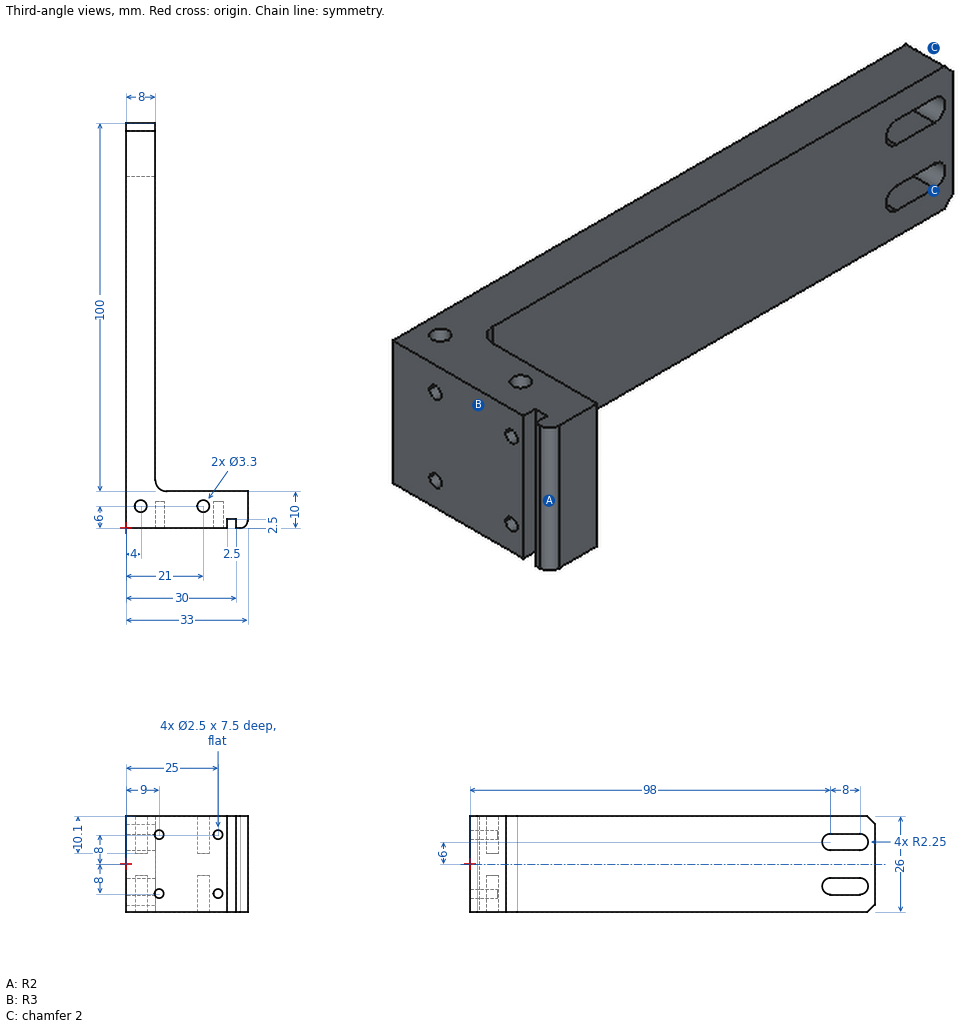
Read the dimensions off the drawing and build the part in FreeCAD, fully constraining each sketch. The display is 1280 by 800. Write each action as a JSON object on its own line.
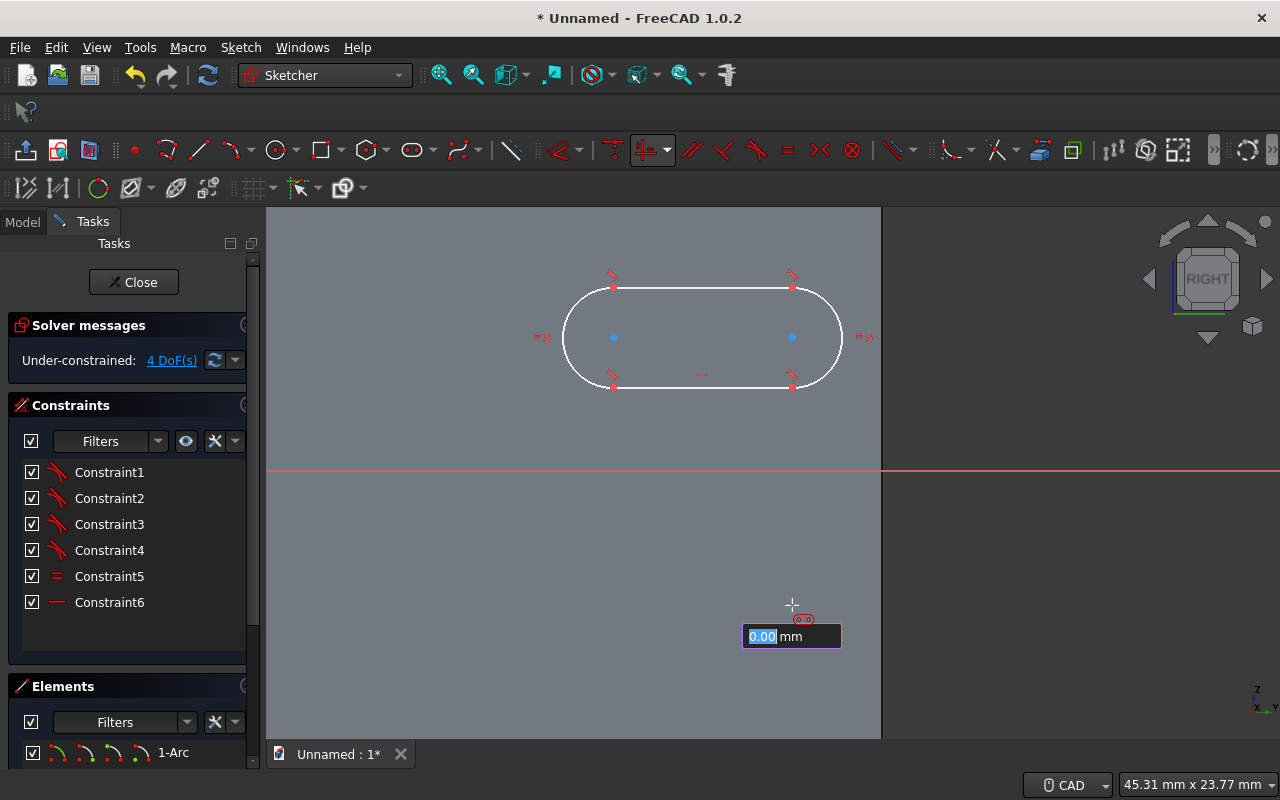
{"action": "left_click", "coordinate": [703, 555]}
{"action": "key", "text": "Escape"}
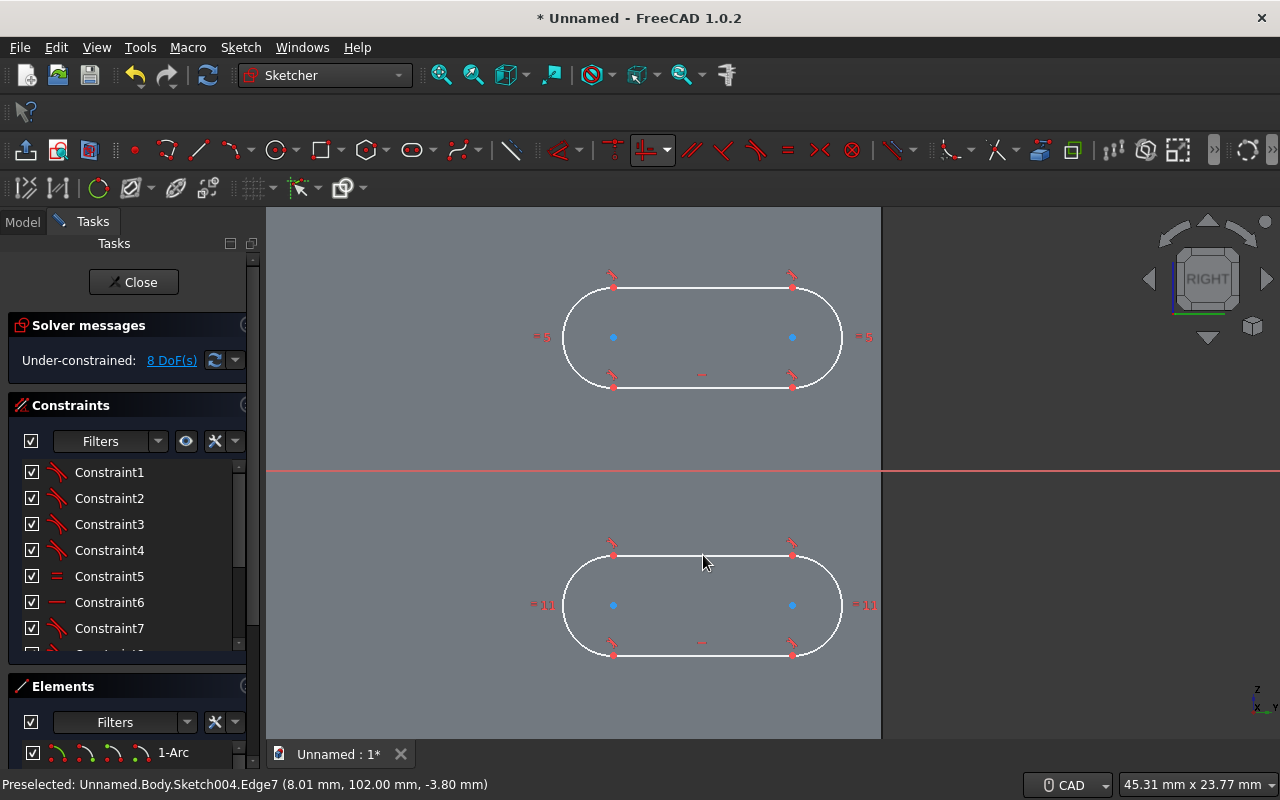
{"action": "left_click", "coordinate": [573, 309]}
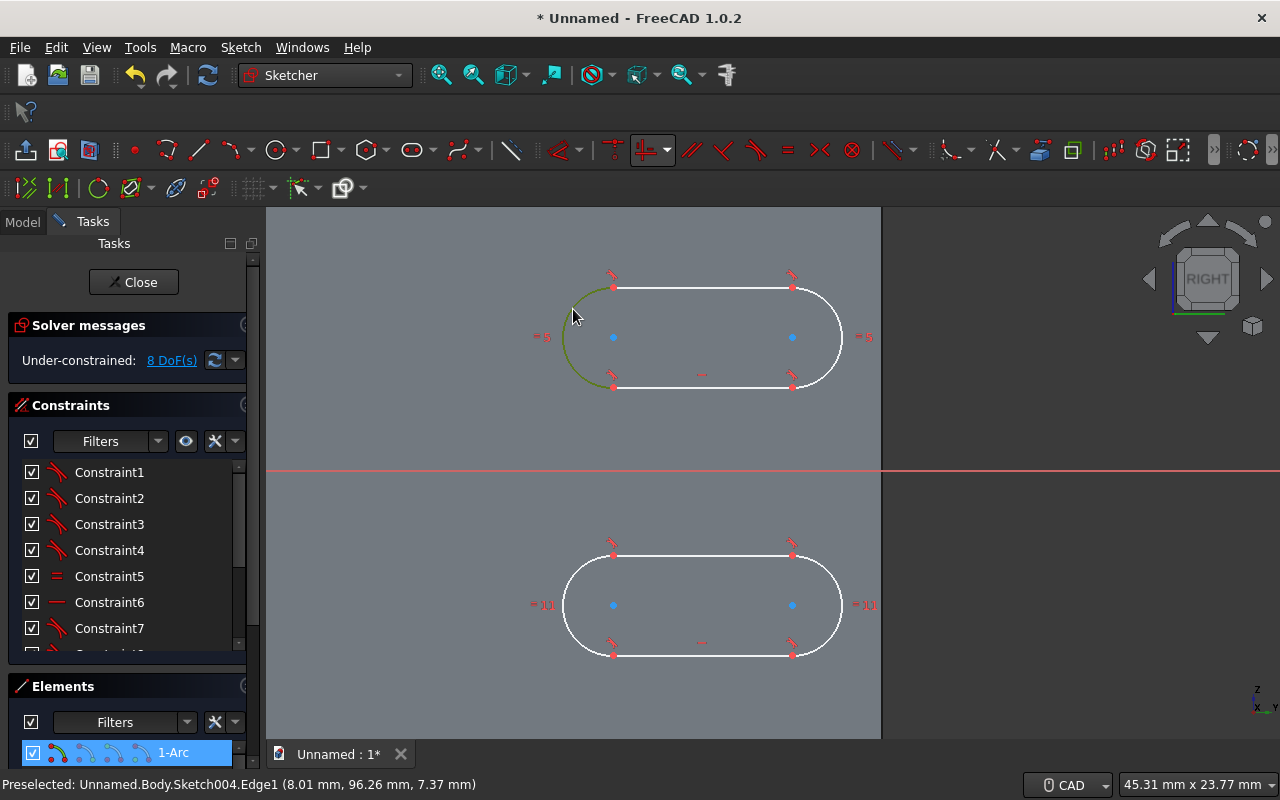
{"action": "left_click", "coordinate": [573, 577]}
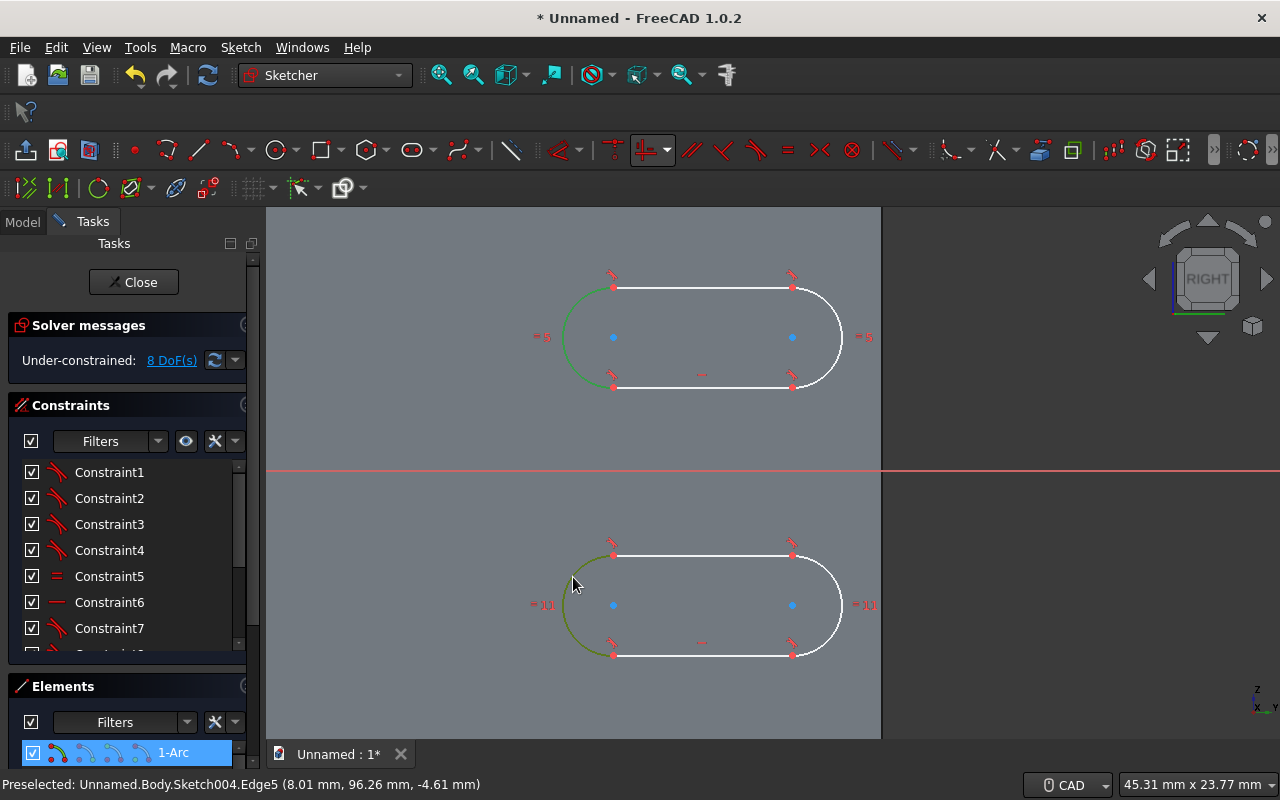
{"action": "left_click", "coordinate": [788, 150]}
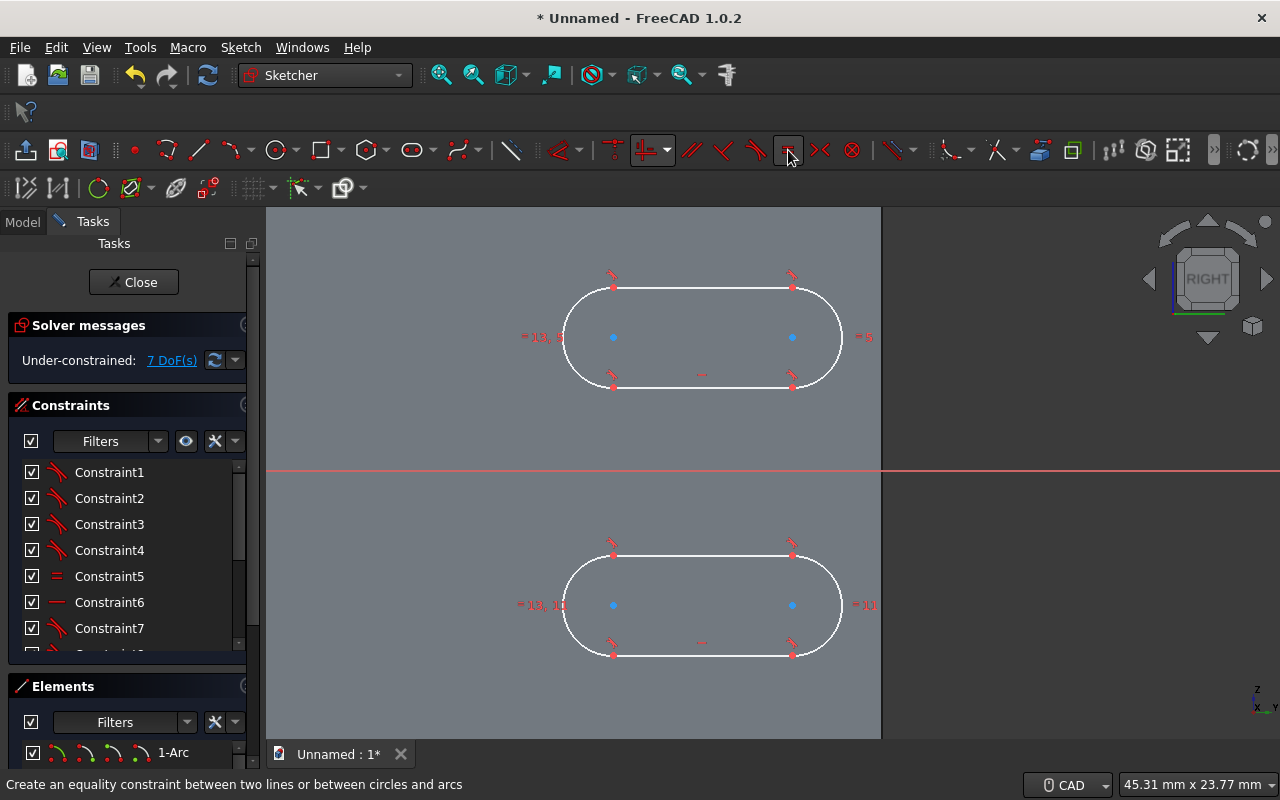
{"action": "left_click", "coordinate": [613, 338]}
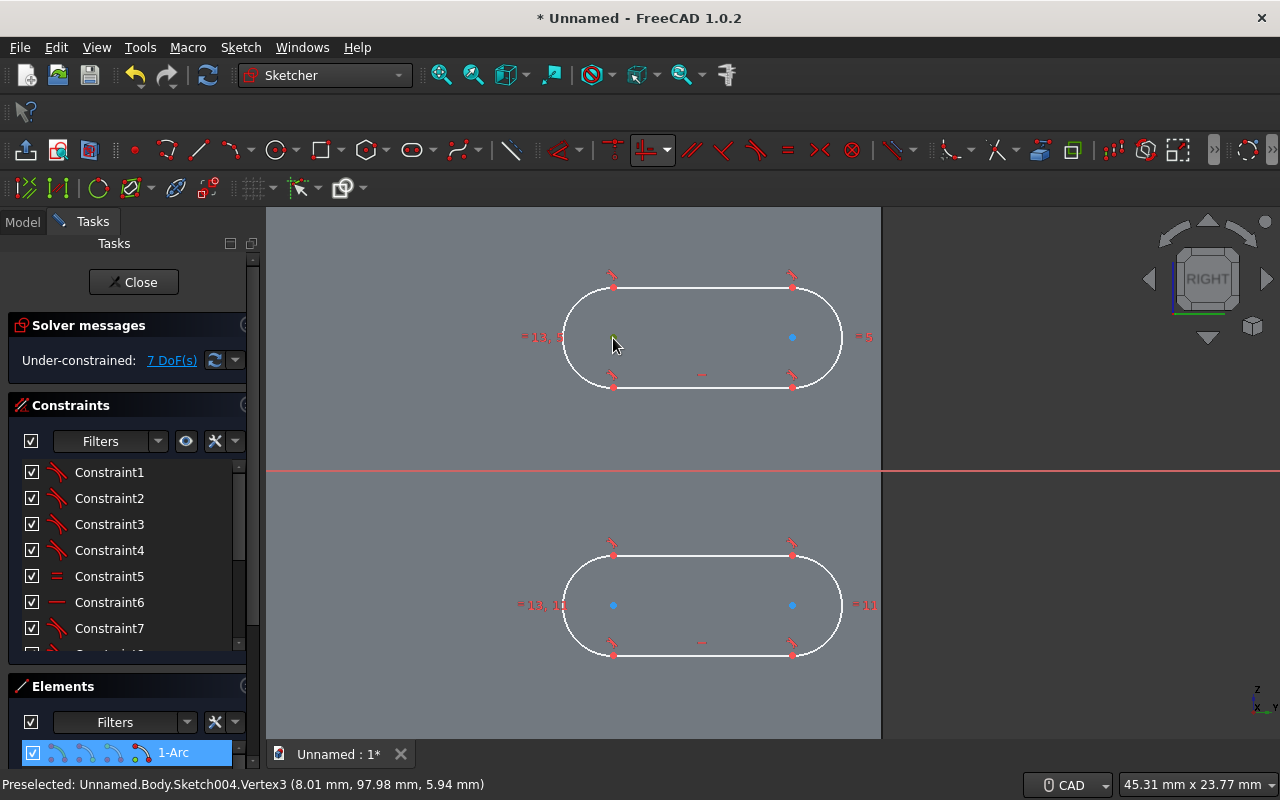
{"action": "left_click", "coordinate": [613, 606]}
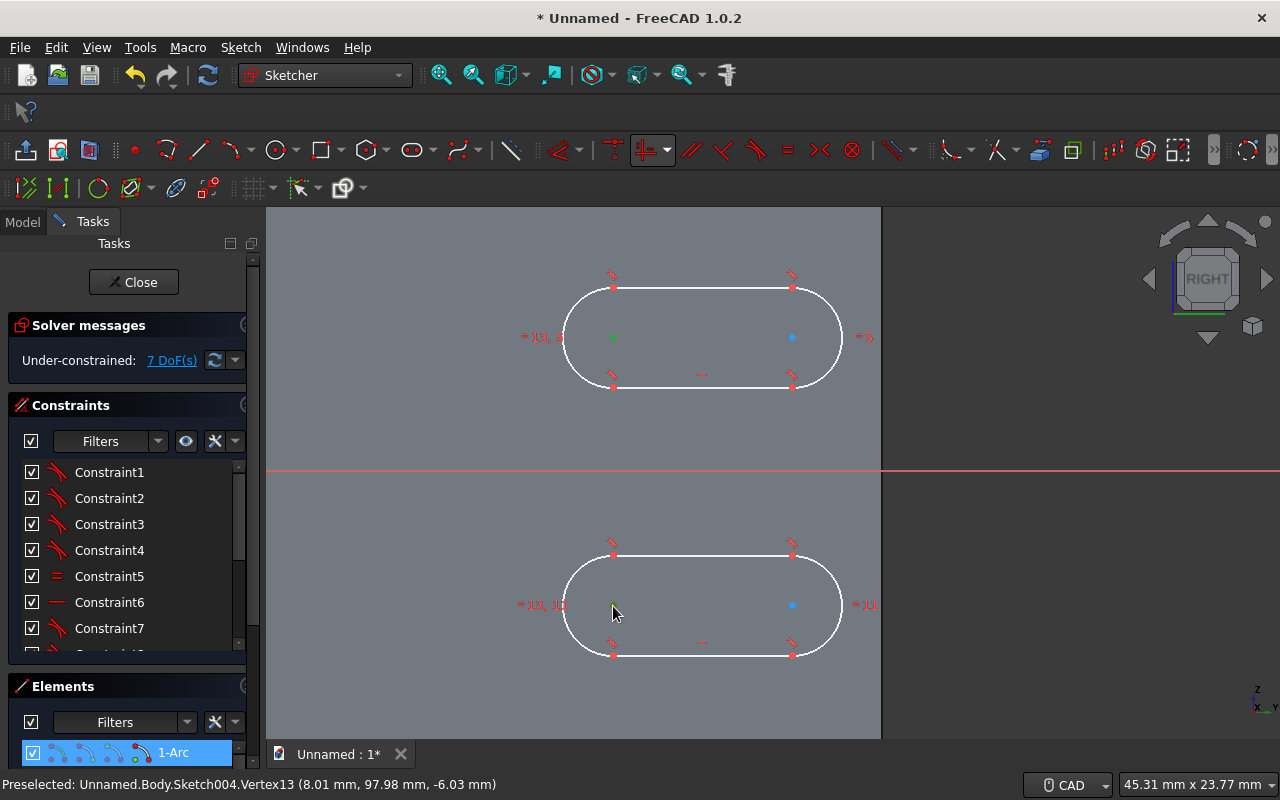
{"action": "left_click", "coordinate": [353, 471]}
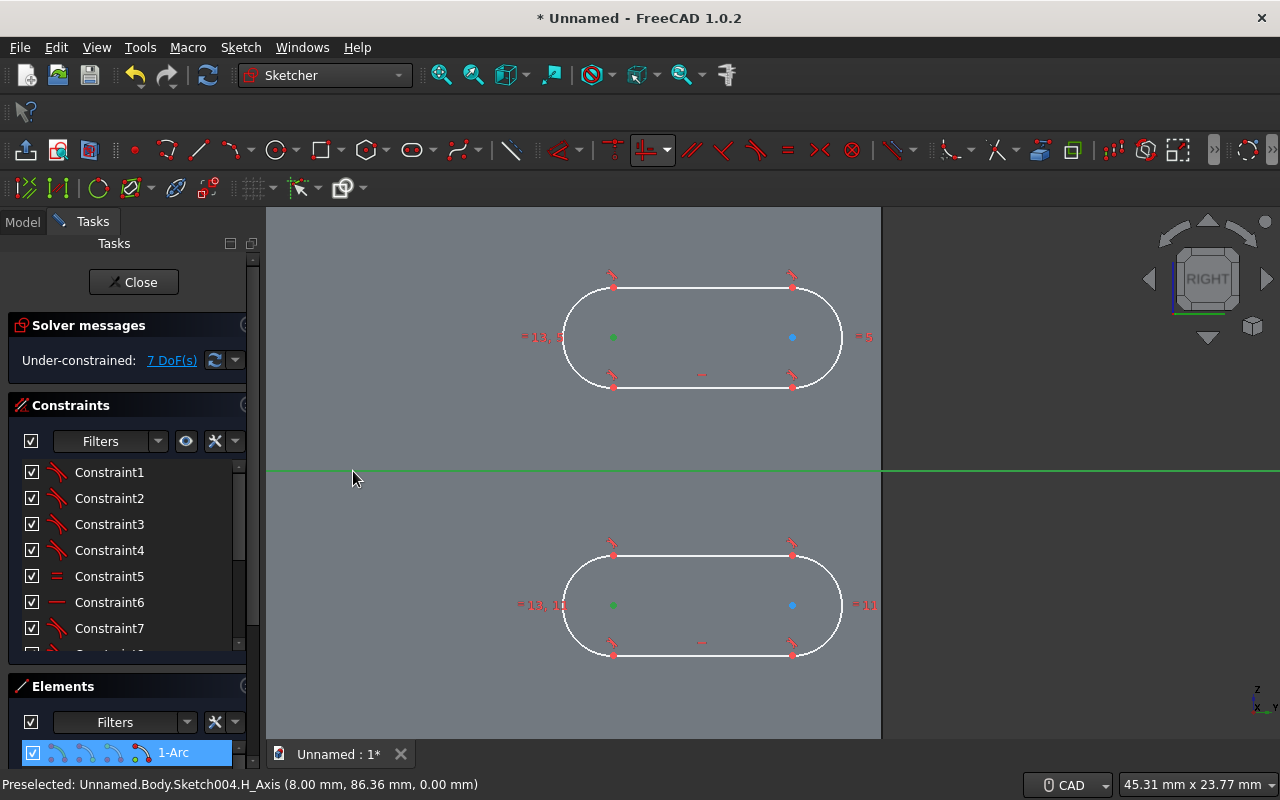
{"action": "left_click", "coordinate": [820, 150]}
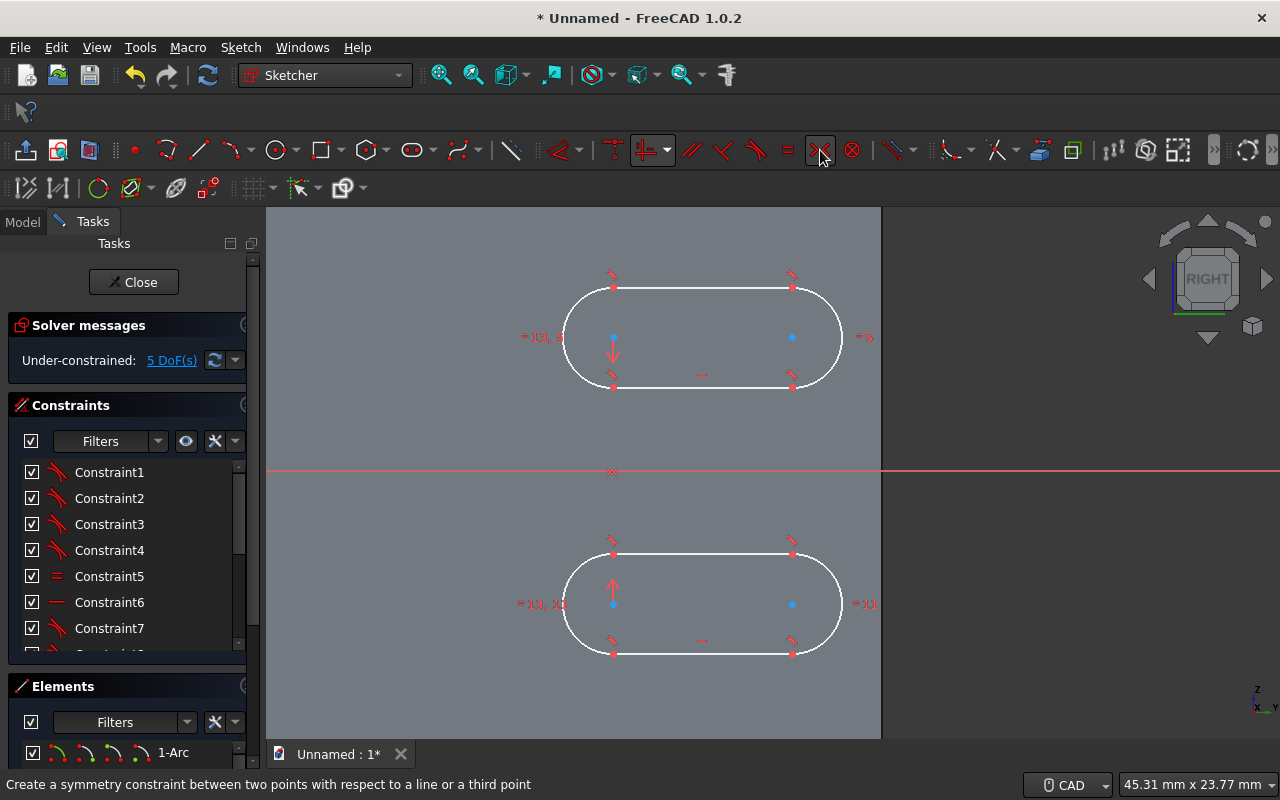
{"action": "left_click", "coordinate": [558, 150]}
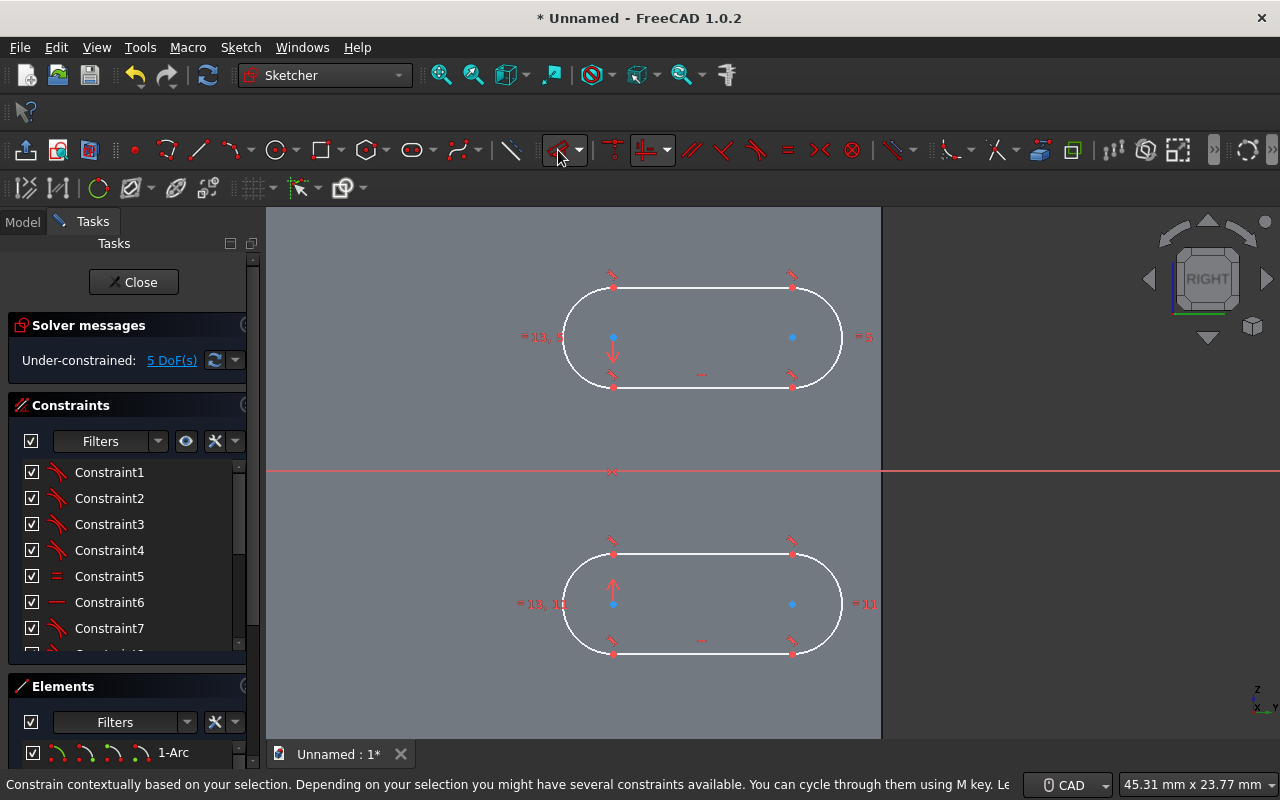
{"action": "left_click", "coordinate": [573, 309]}
{"action": "left_click", "coordinate": [547, 290]}